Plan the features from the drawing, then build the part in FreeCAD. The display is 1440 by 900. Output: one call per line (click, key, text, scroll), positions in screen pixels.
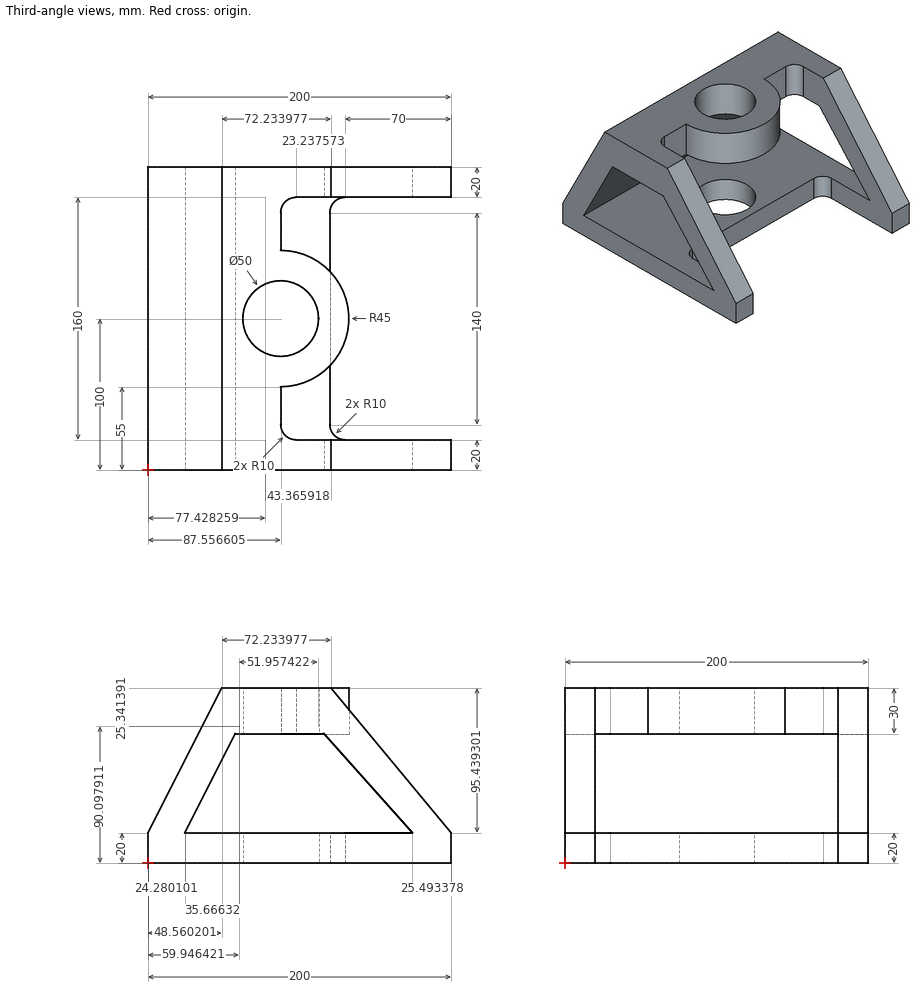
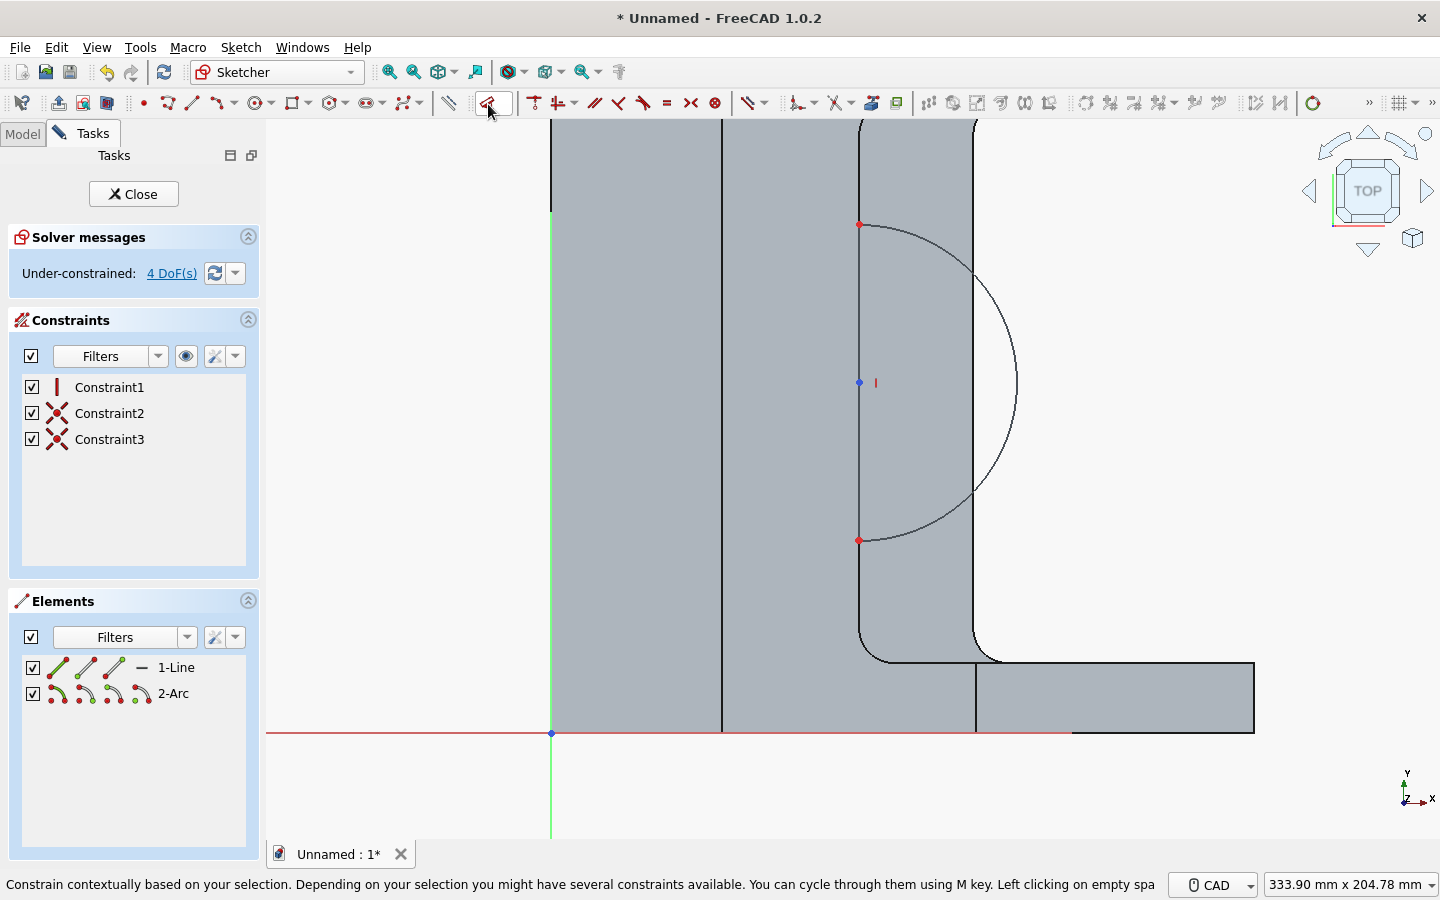
click(987, 476)
click(1013, 495)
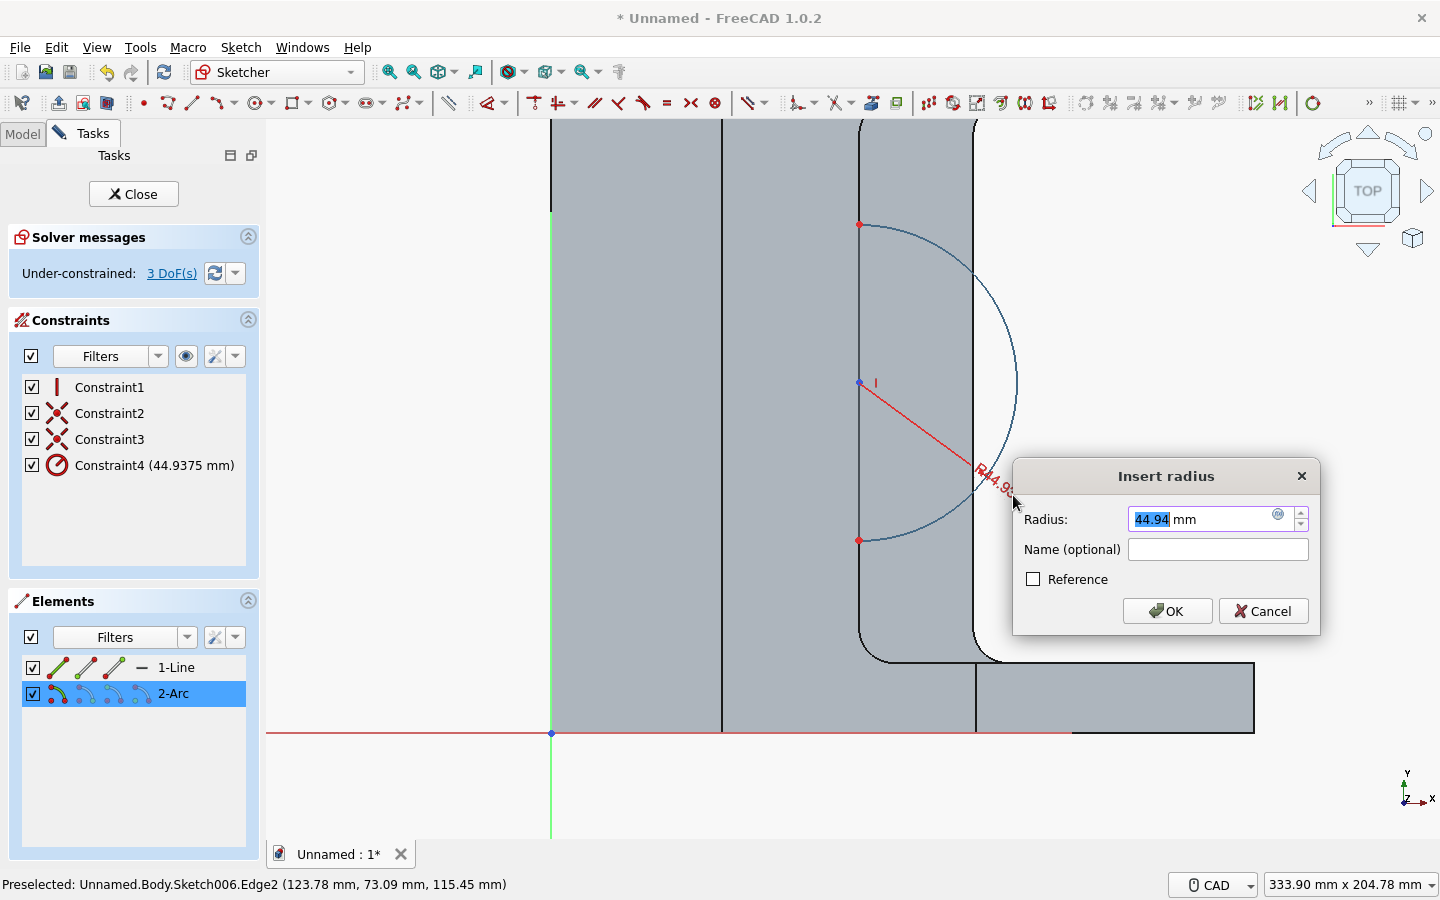
text(45)
key(Return)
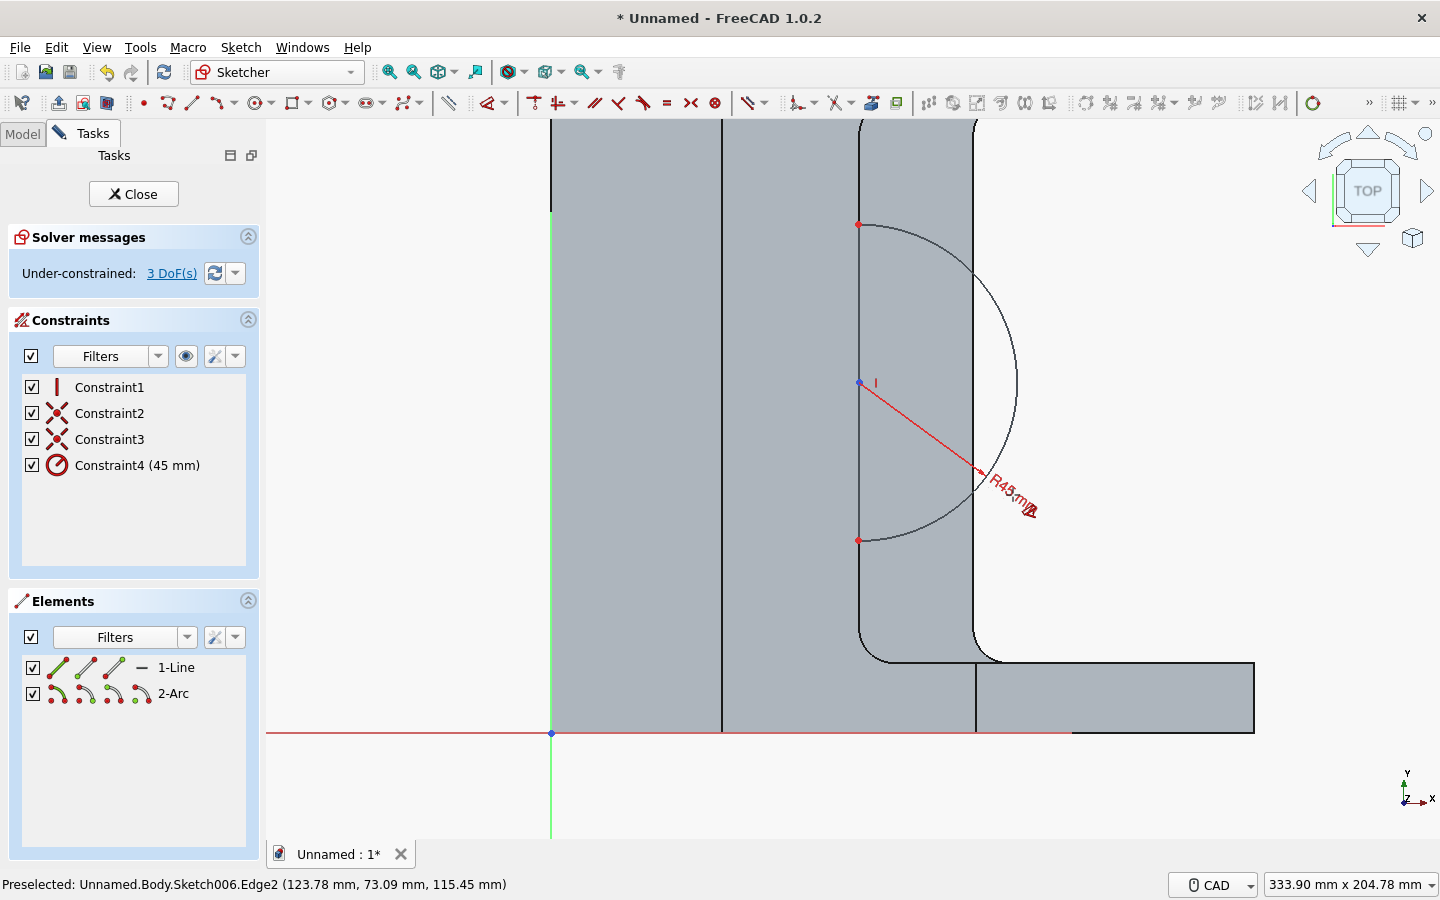
click(859, 541)
click(517, 637)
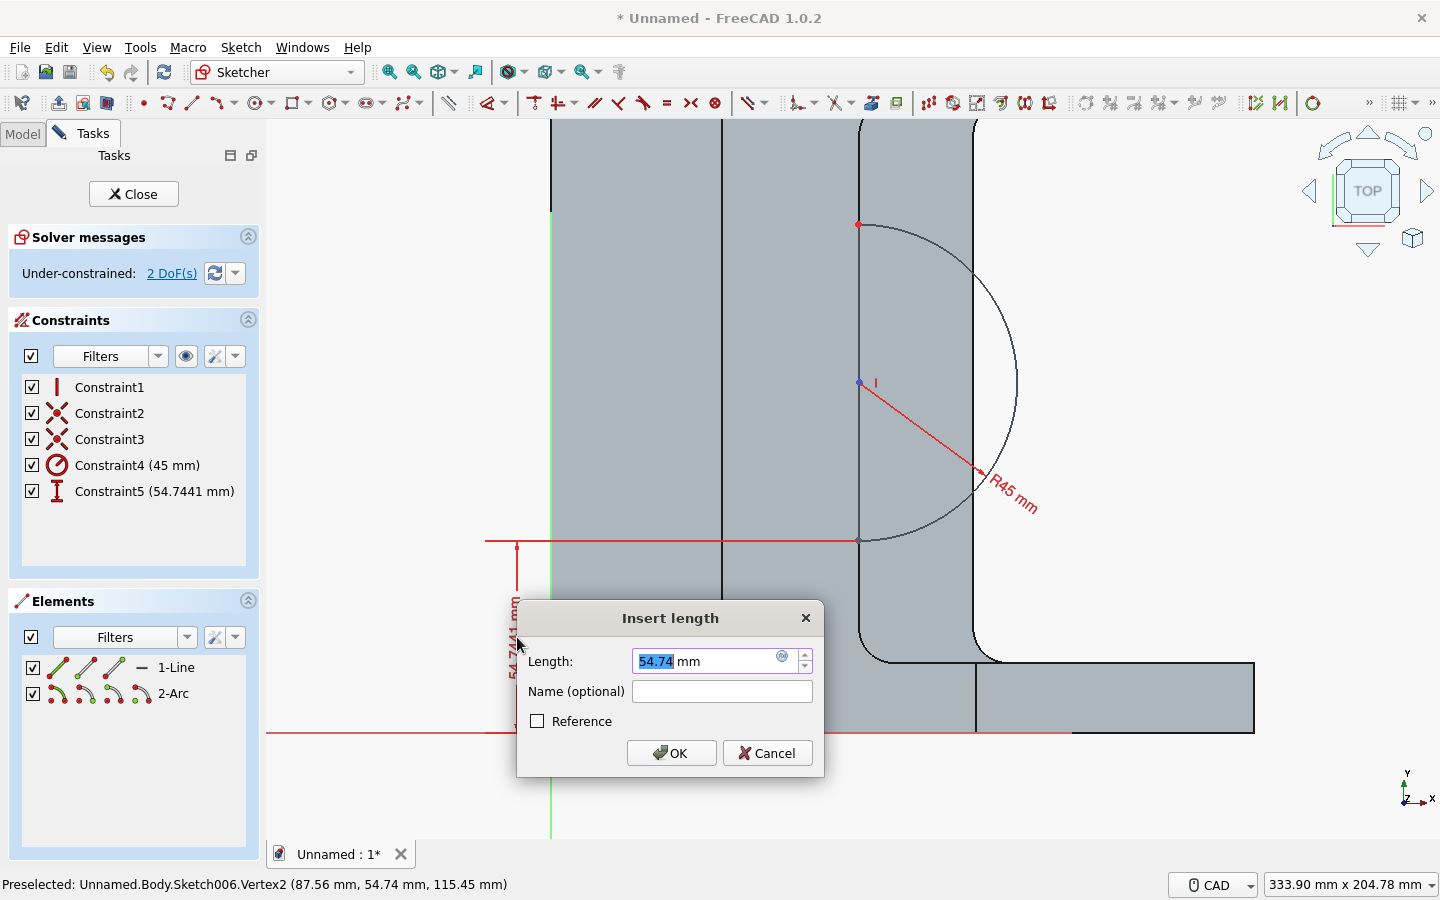
text(55)
key(Return)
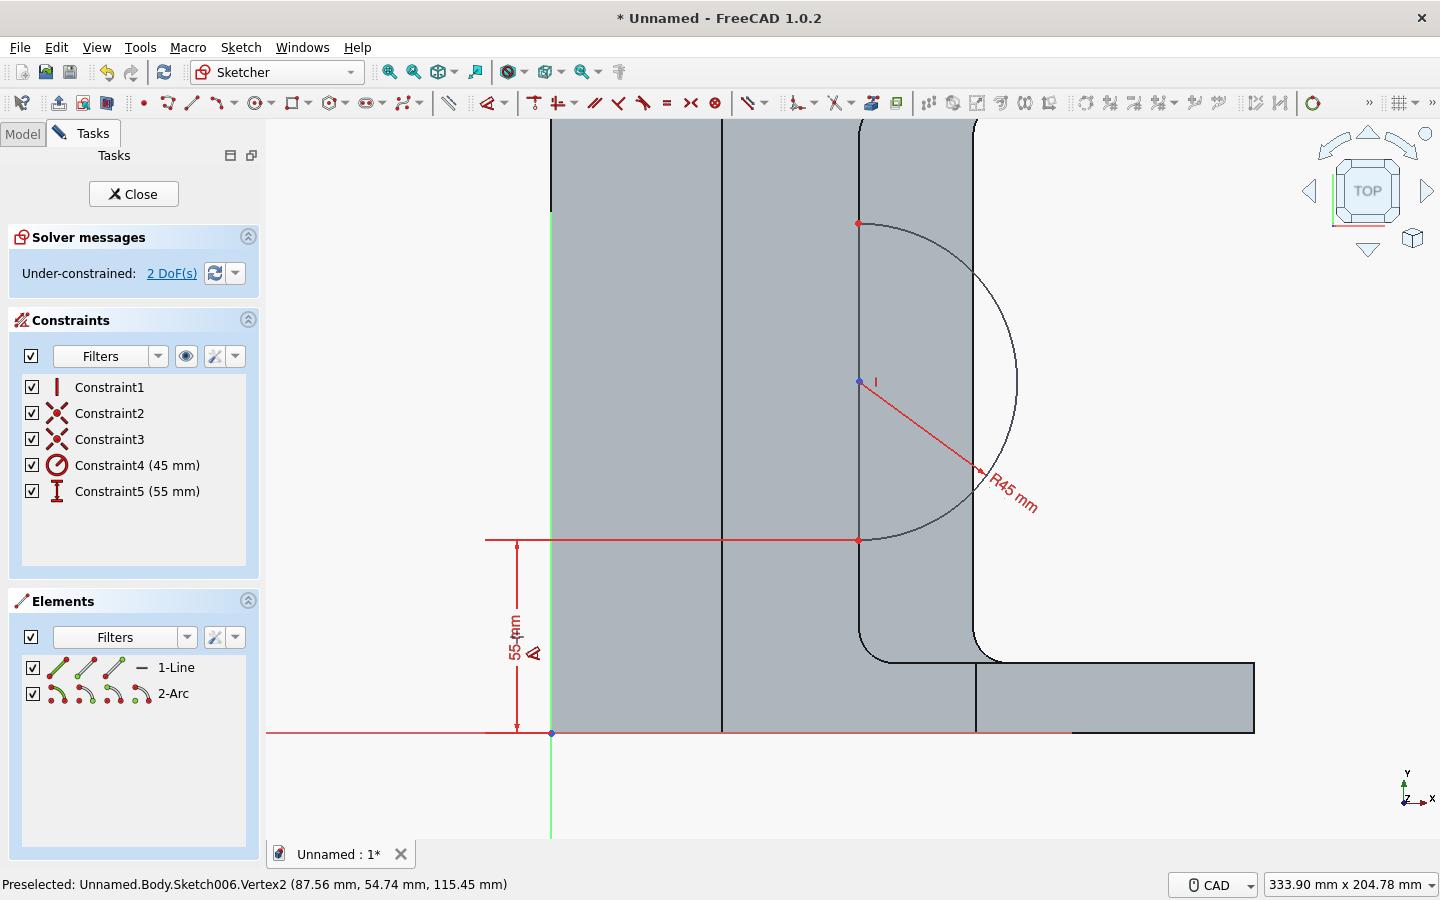
click(859, 224)
click(705, 767)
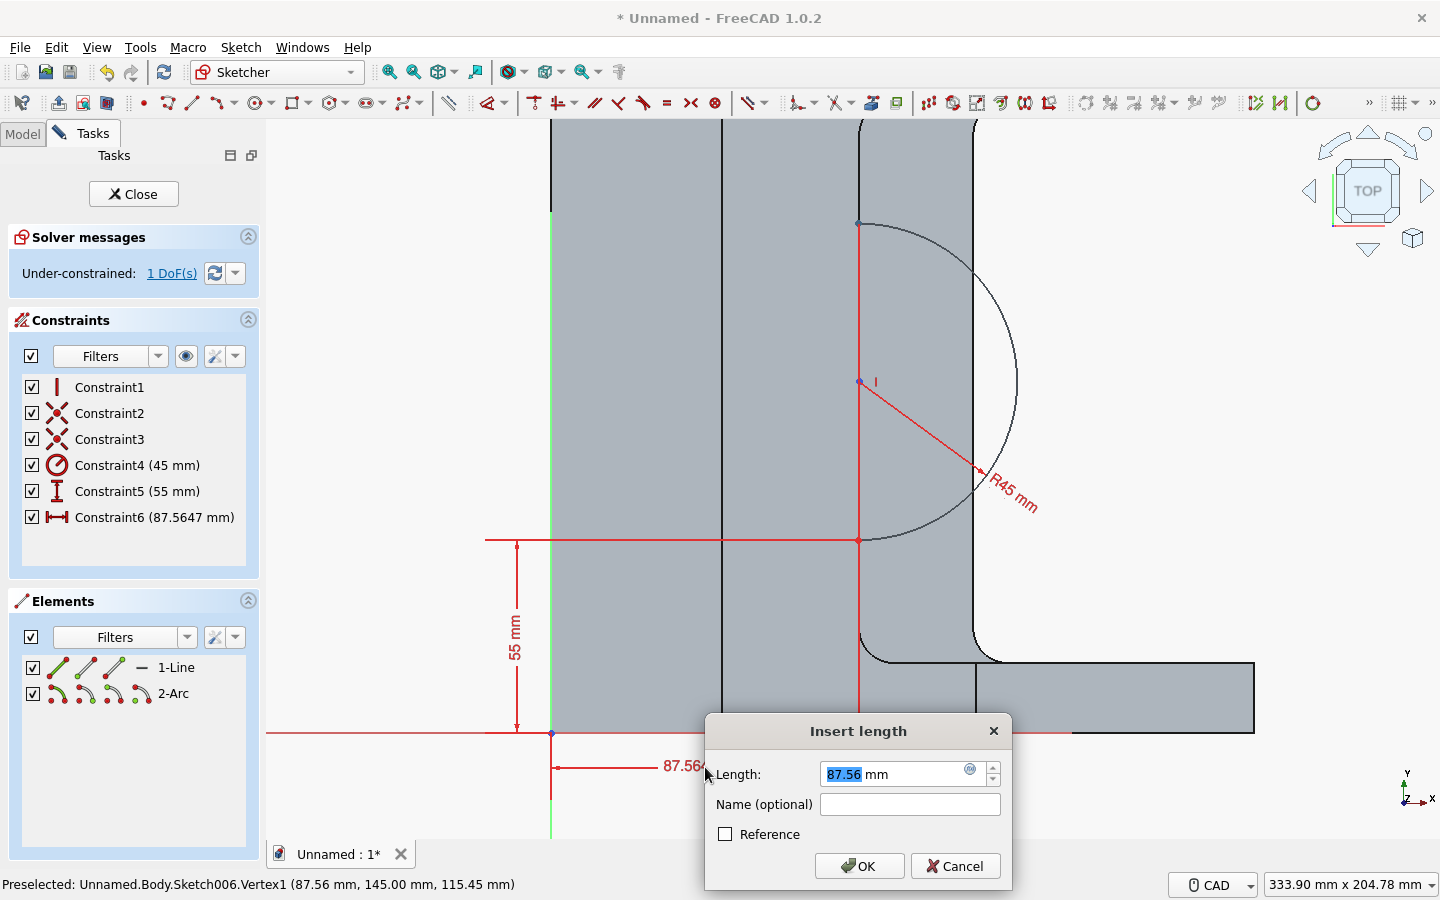
text(87.556605)
key(Return)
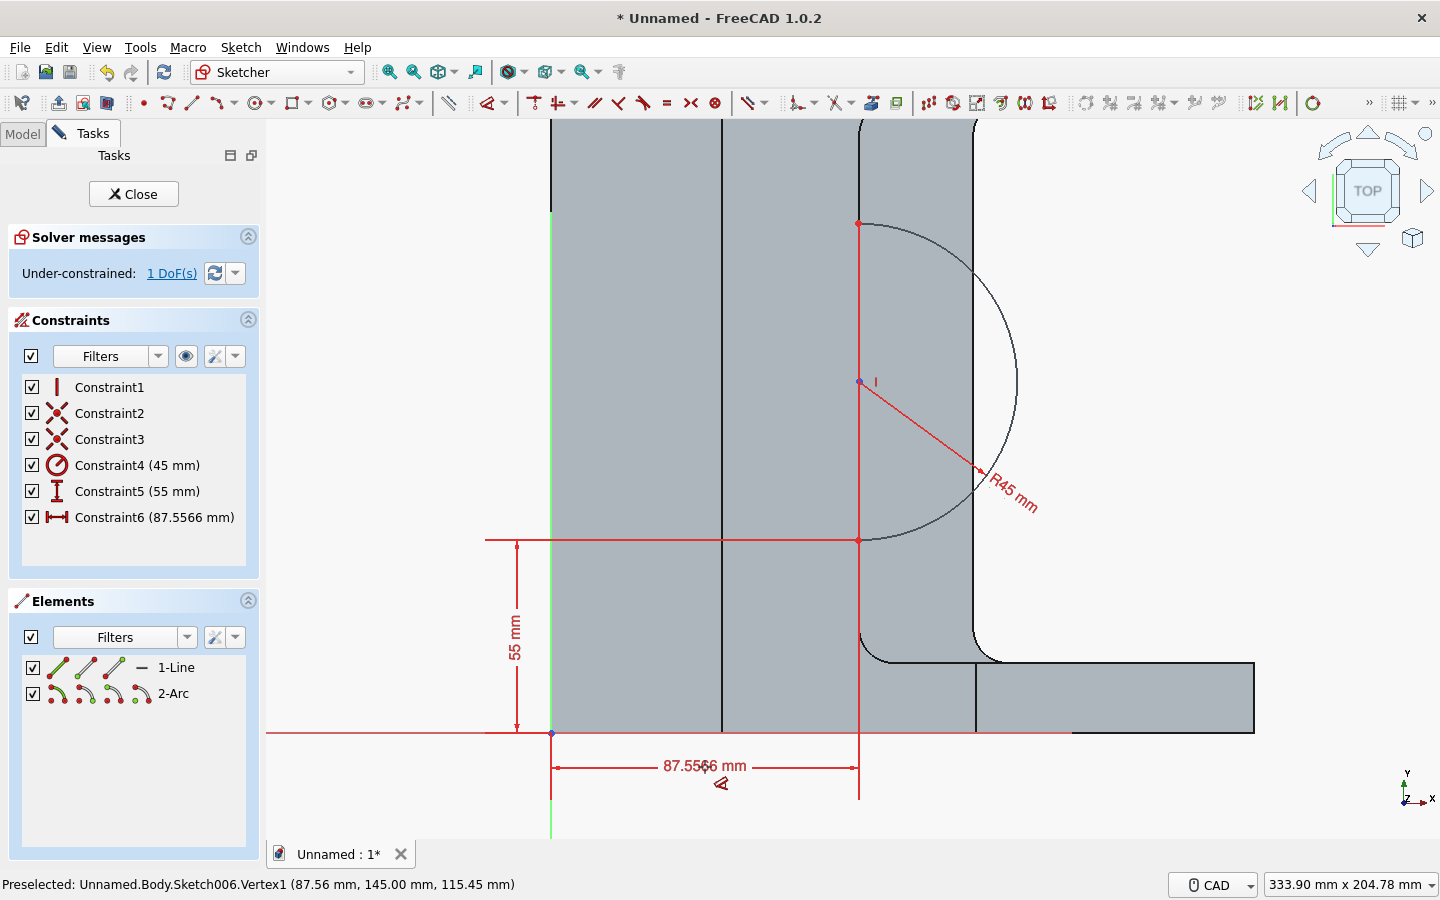
click(859, 382)
click(634, 767)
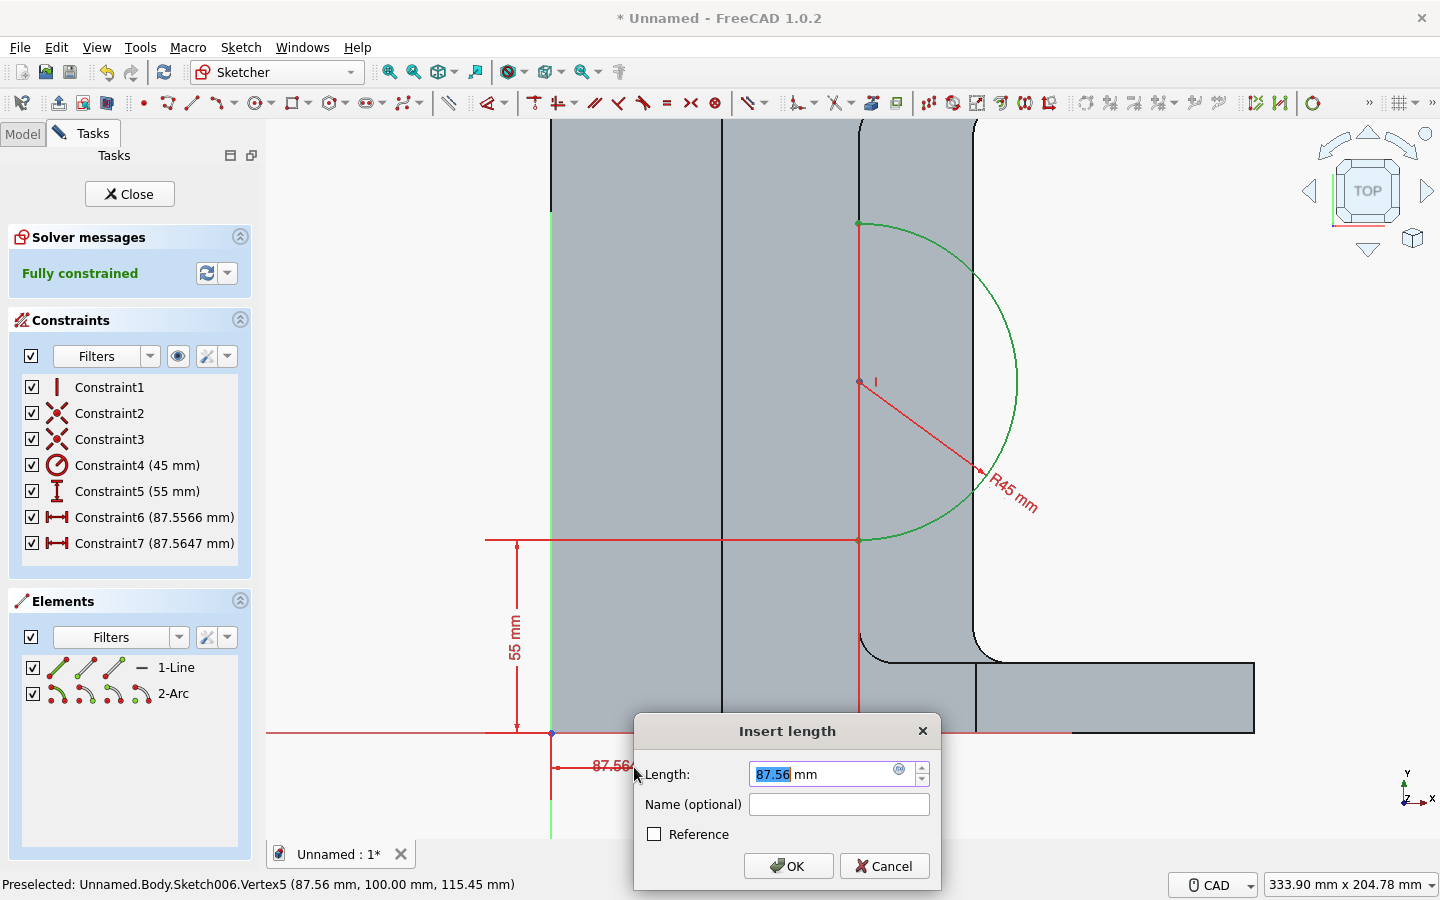
text(87.556605)
key(Return)
key(Escape)